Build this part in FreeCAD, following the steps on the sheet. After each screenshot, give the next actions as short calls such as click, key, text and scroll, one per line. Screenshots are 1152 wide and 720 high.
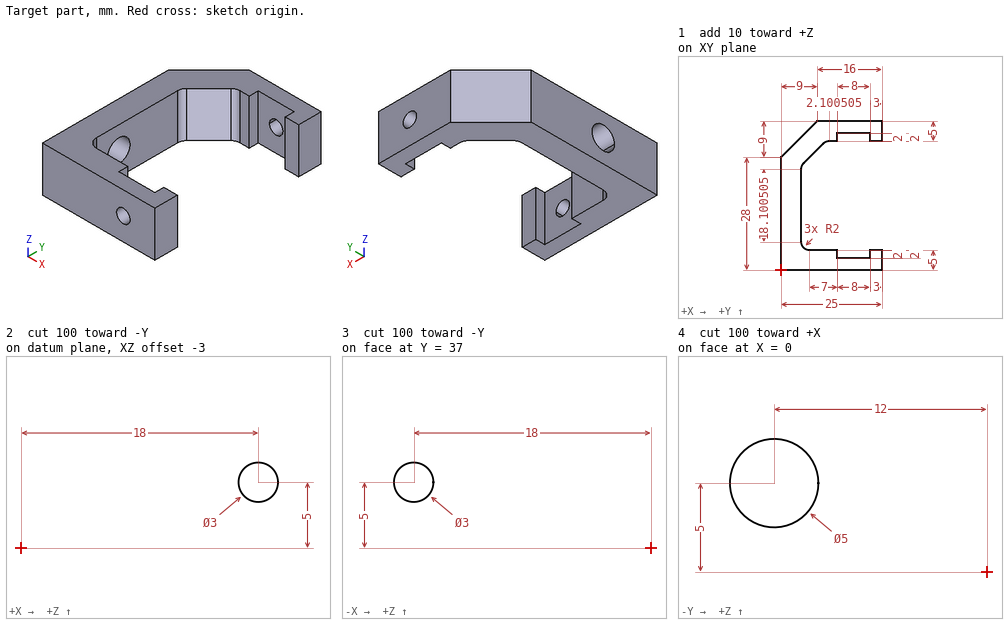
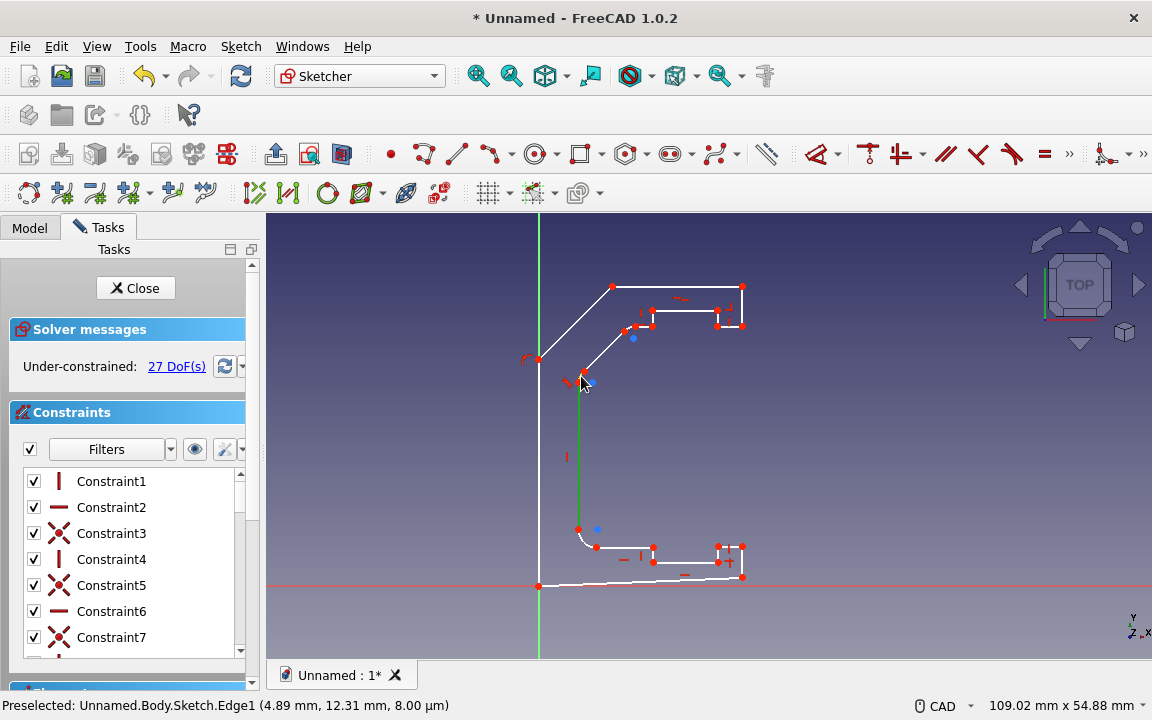
scroll(581, 538, up, 3)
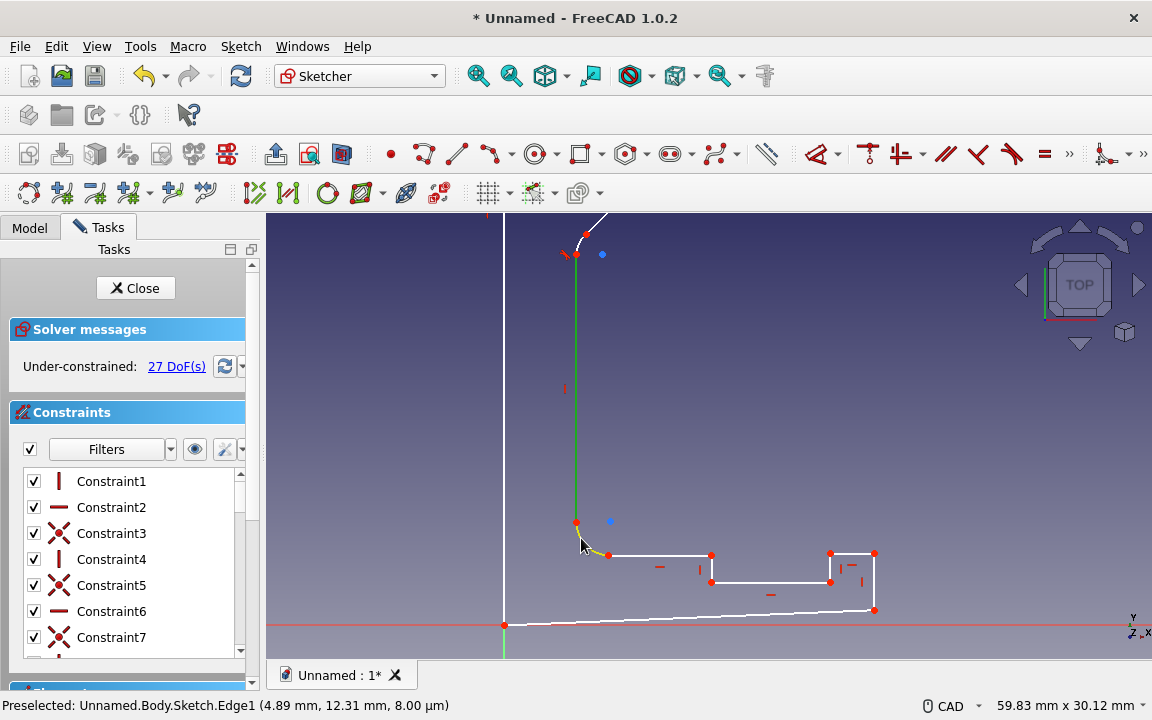
click(580, 537)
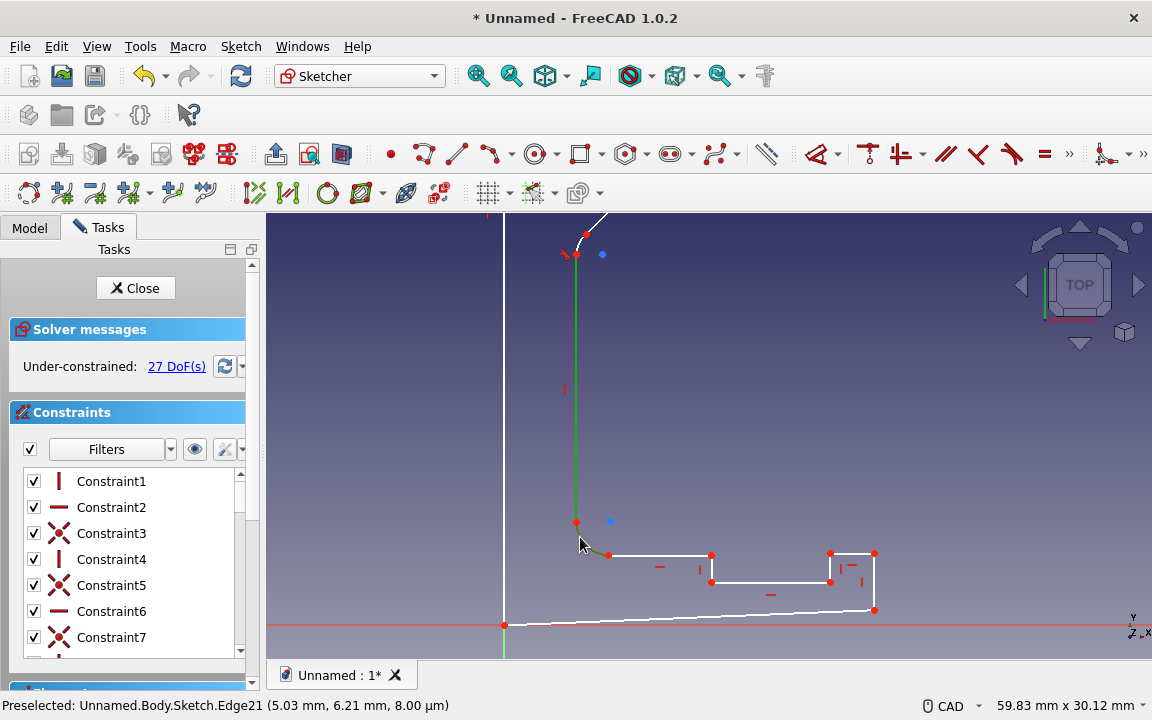
click(1012, 154)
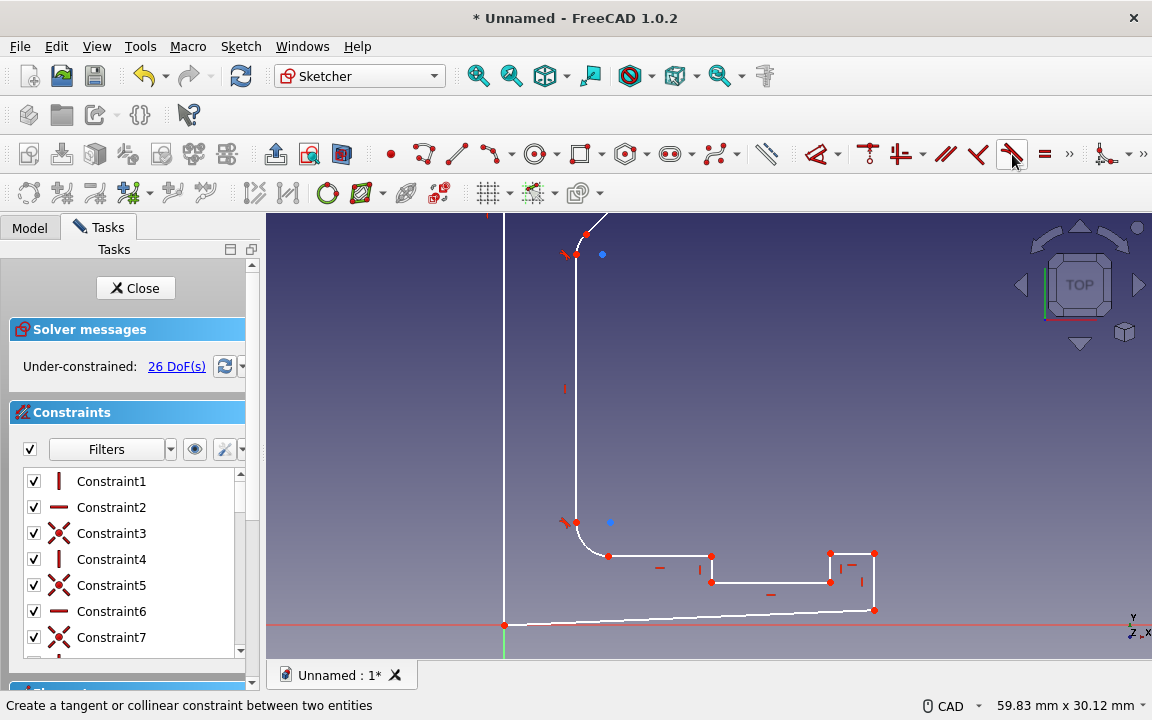
scroll(581, 539, down, 3)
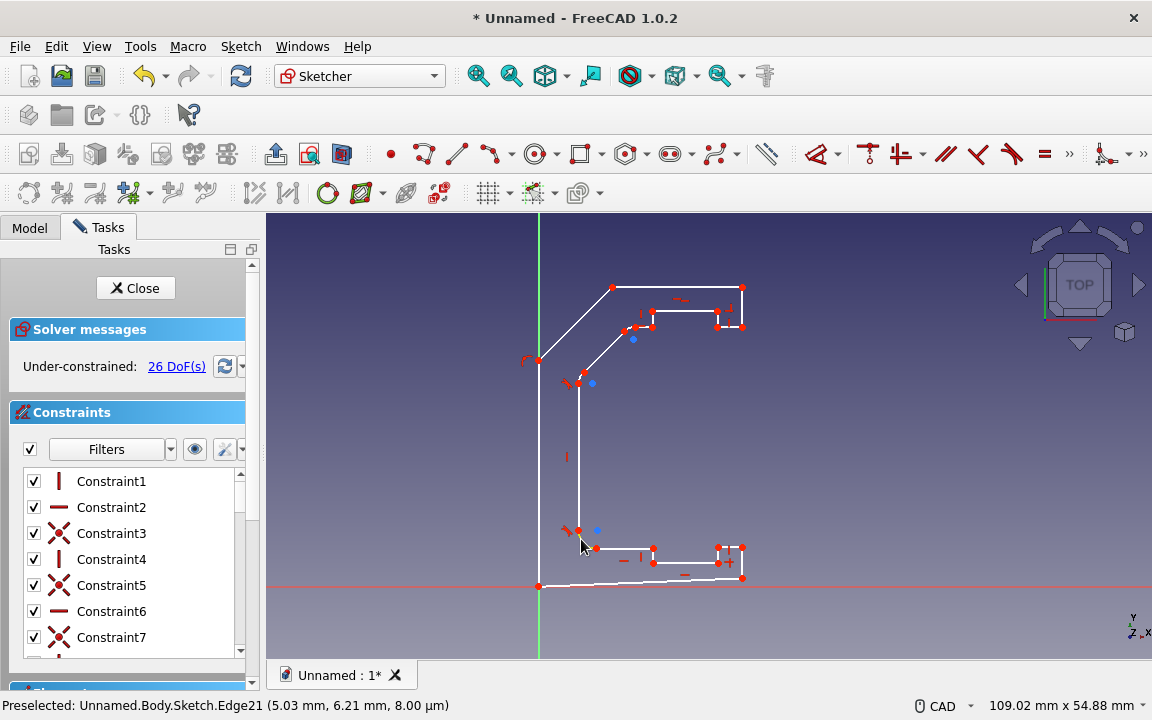
click(596, 360)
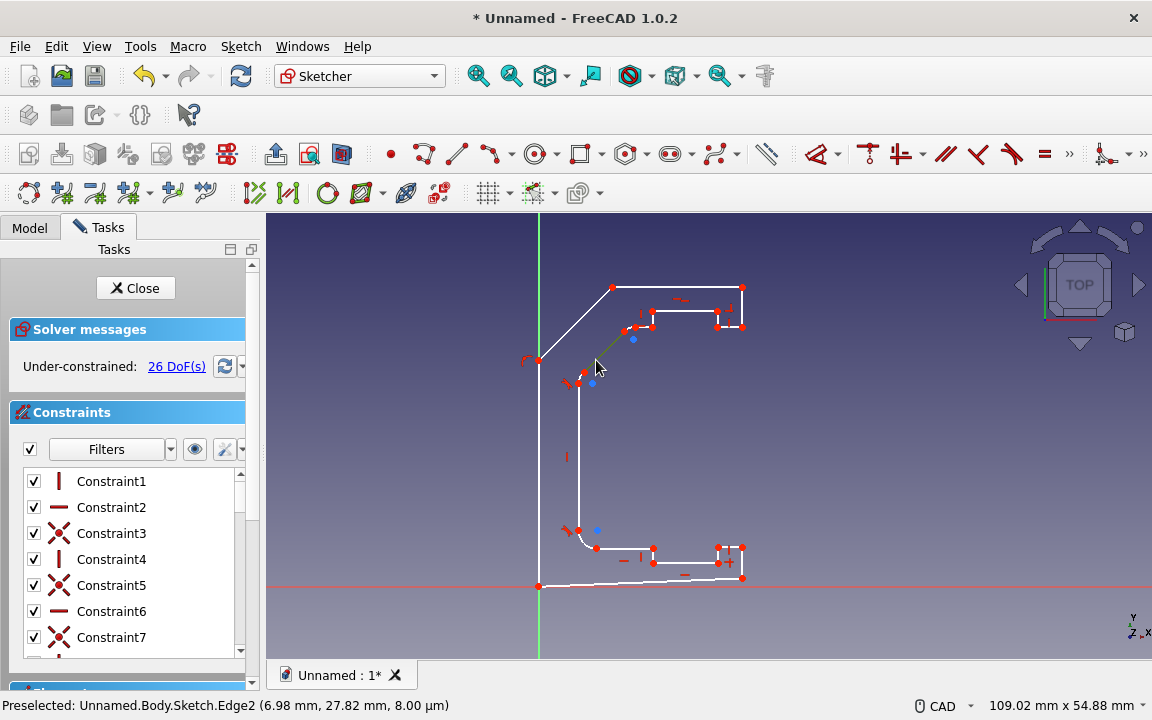
scroll(580, 377, up, 4)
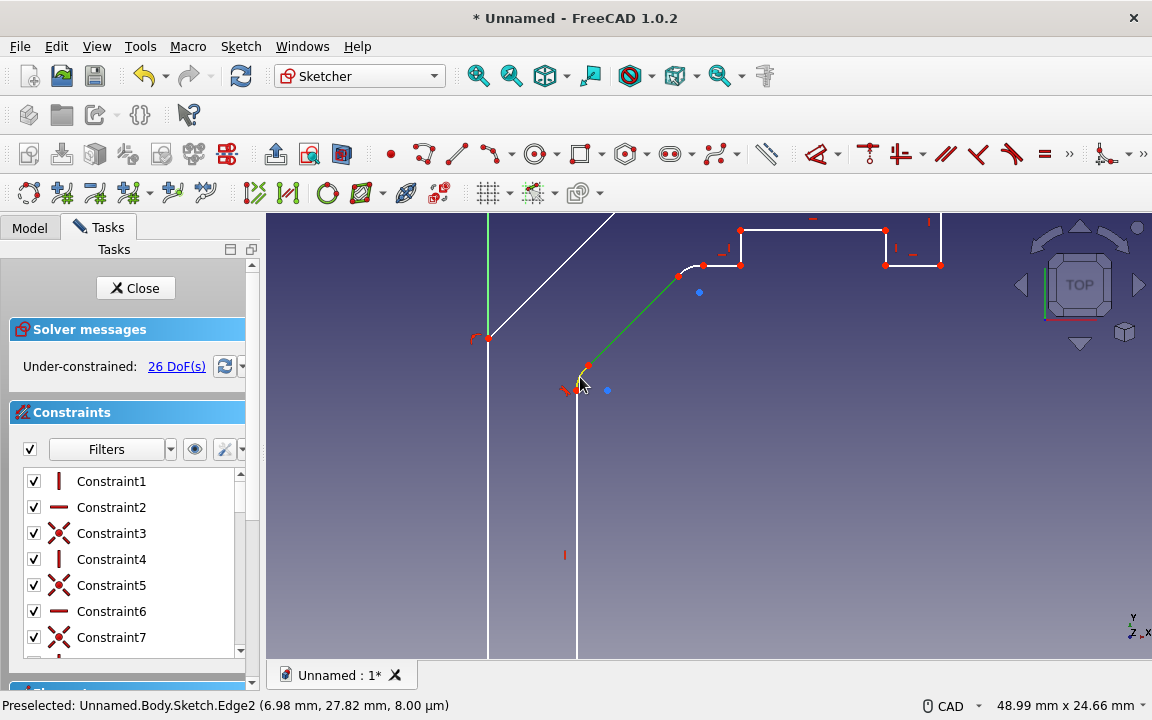
click(580, 377)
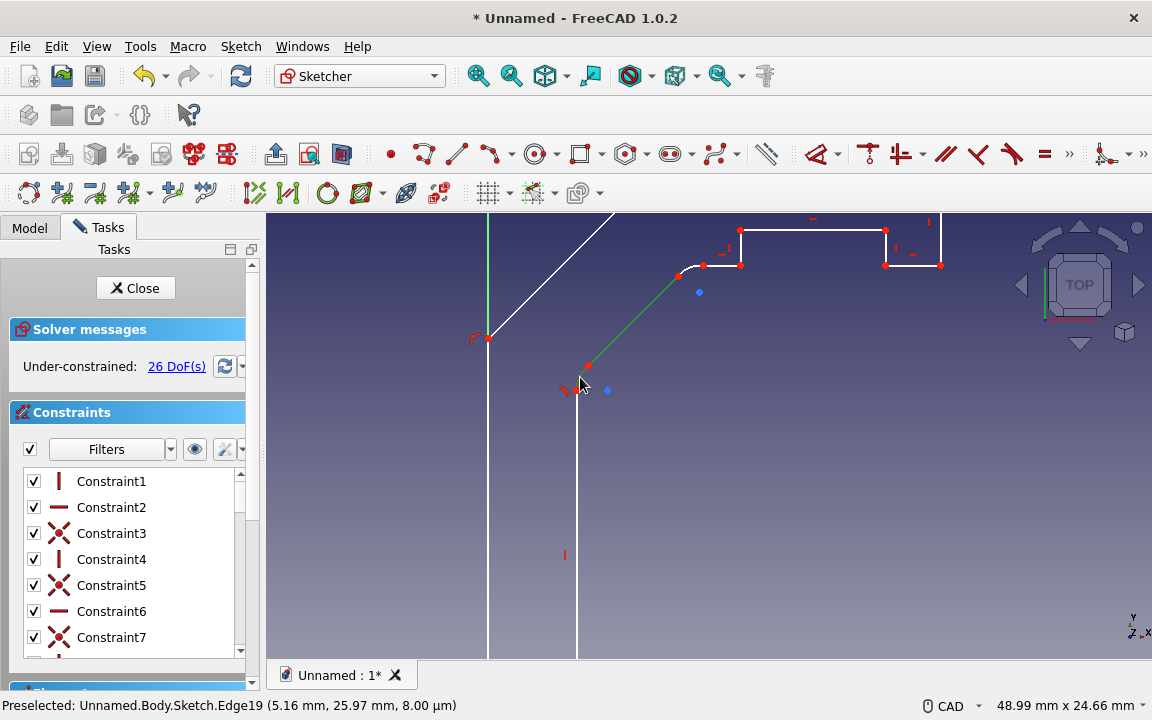
key(t)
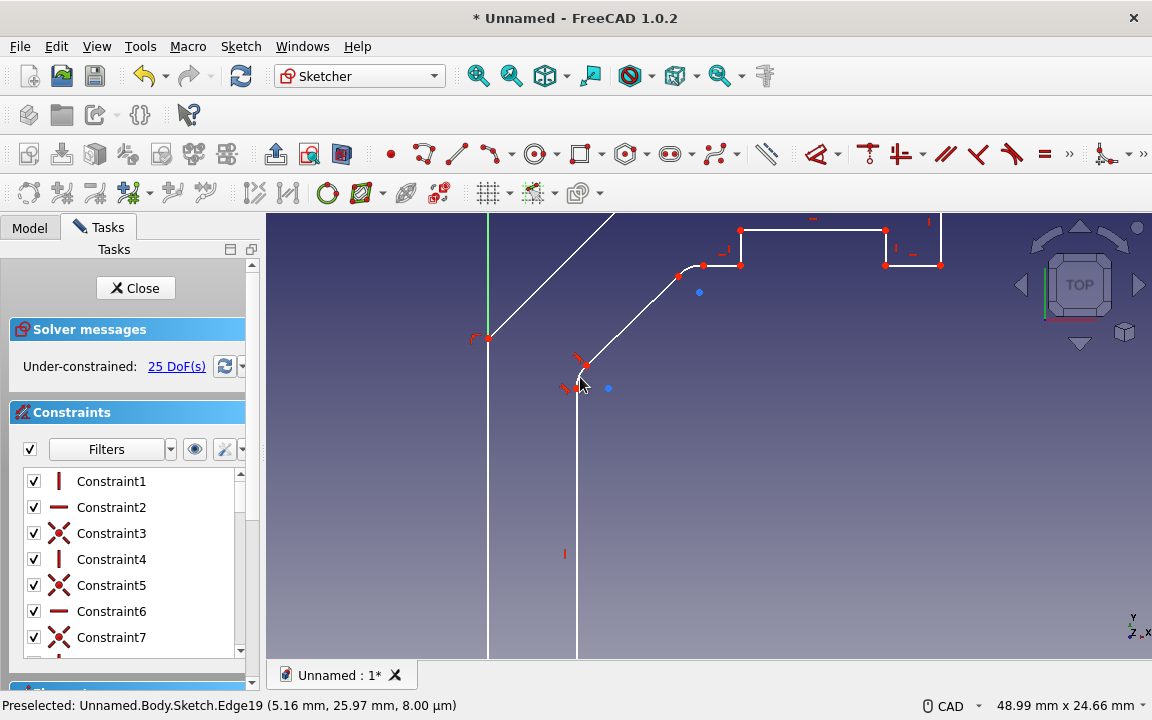
click(614, 339)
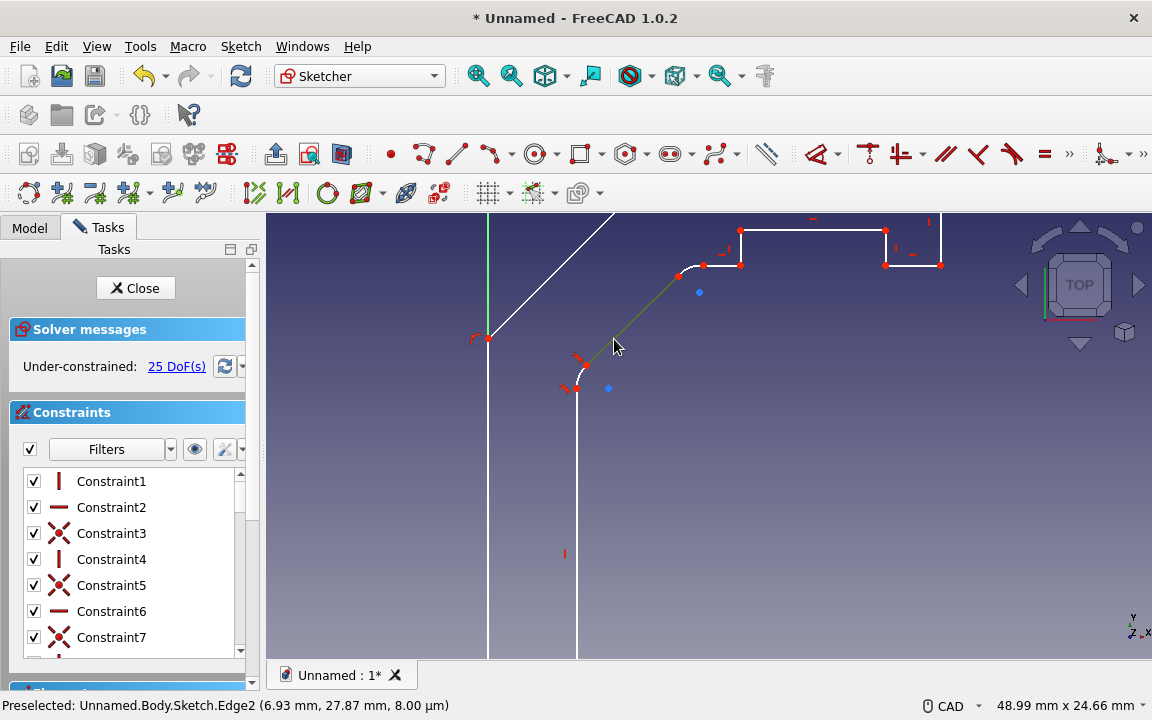
click(690, 268)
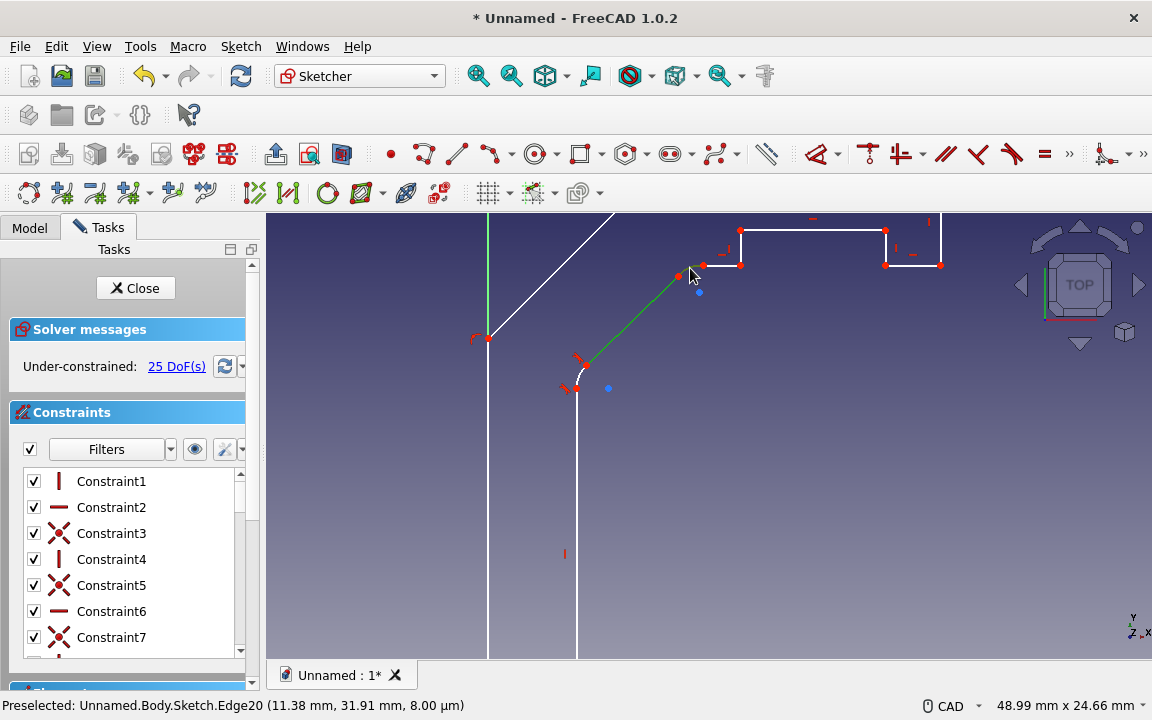
key(t)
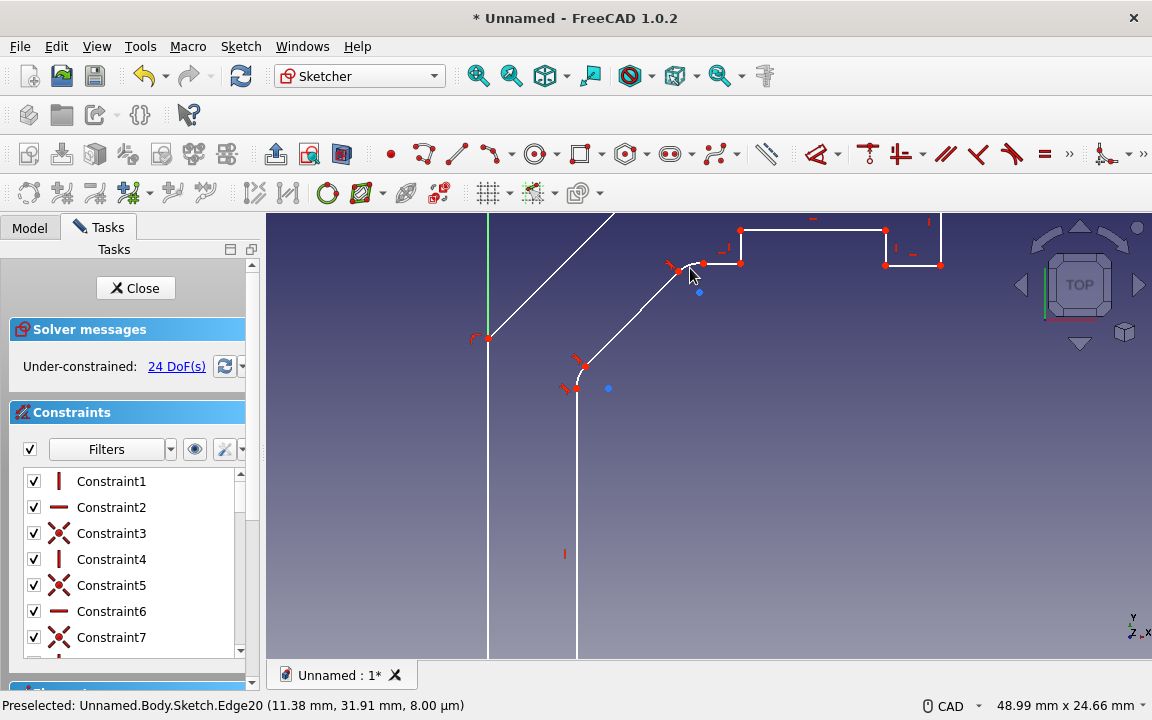
scroll(715, 264, up, 2)